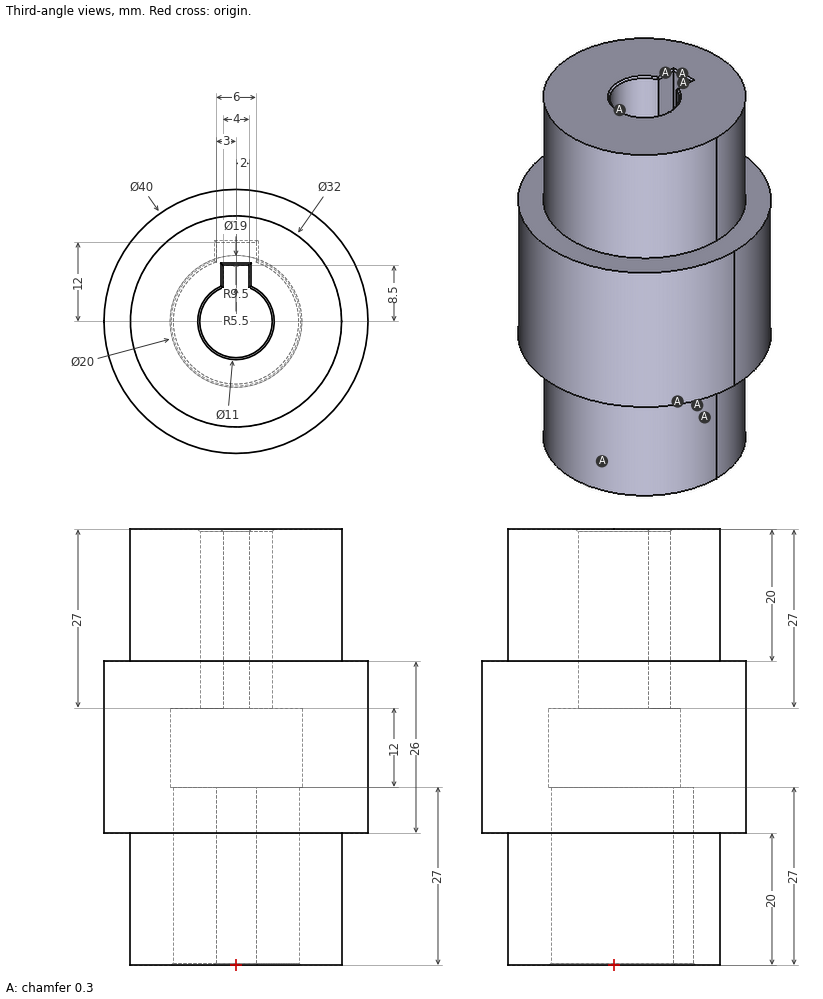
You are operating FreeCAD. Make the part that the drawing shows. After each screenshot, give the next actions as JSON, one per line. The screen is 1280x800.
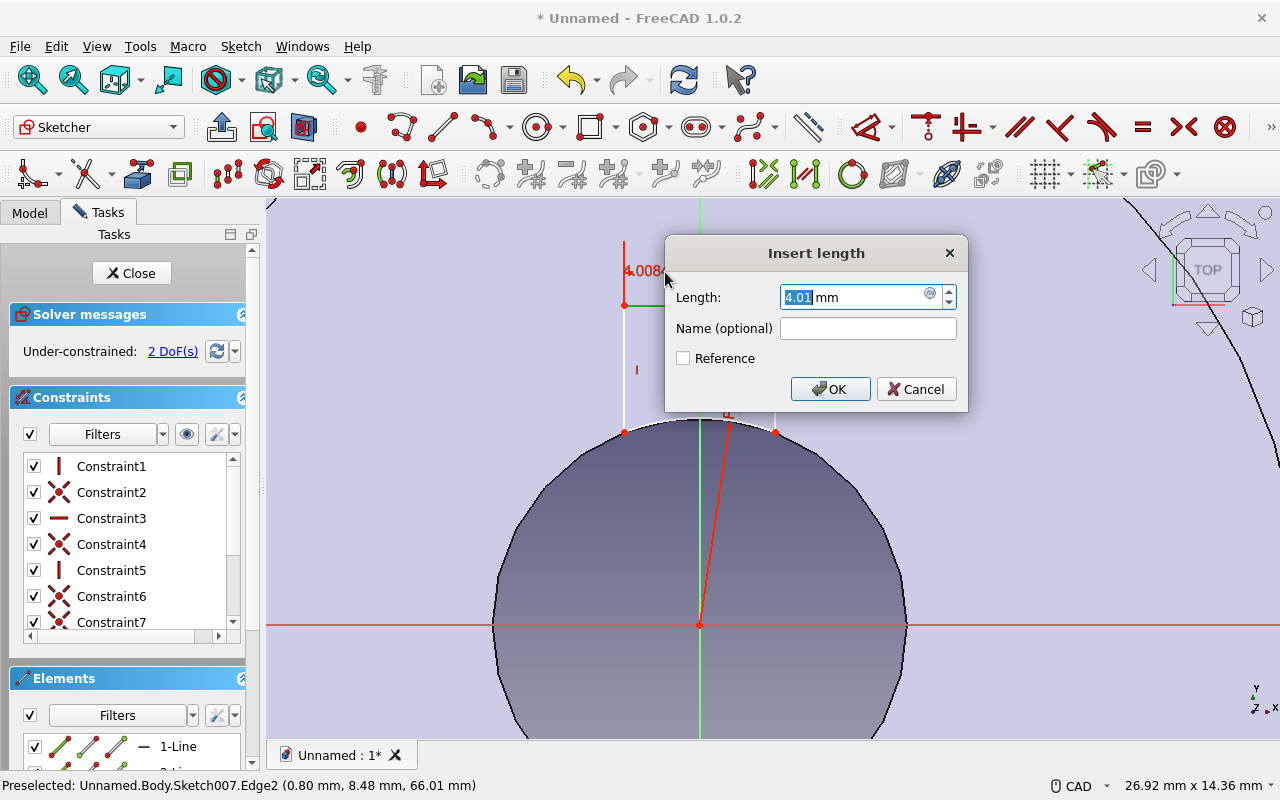
{"action": "type", "text": "4"}
{"action": "key", "text": "Return"}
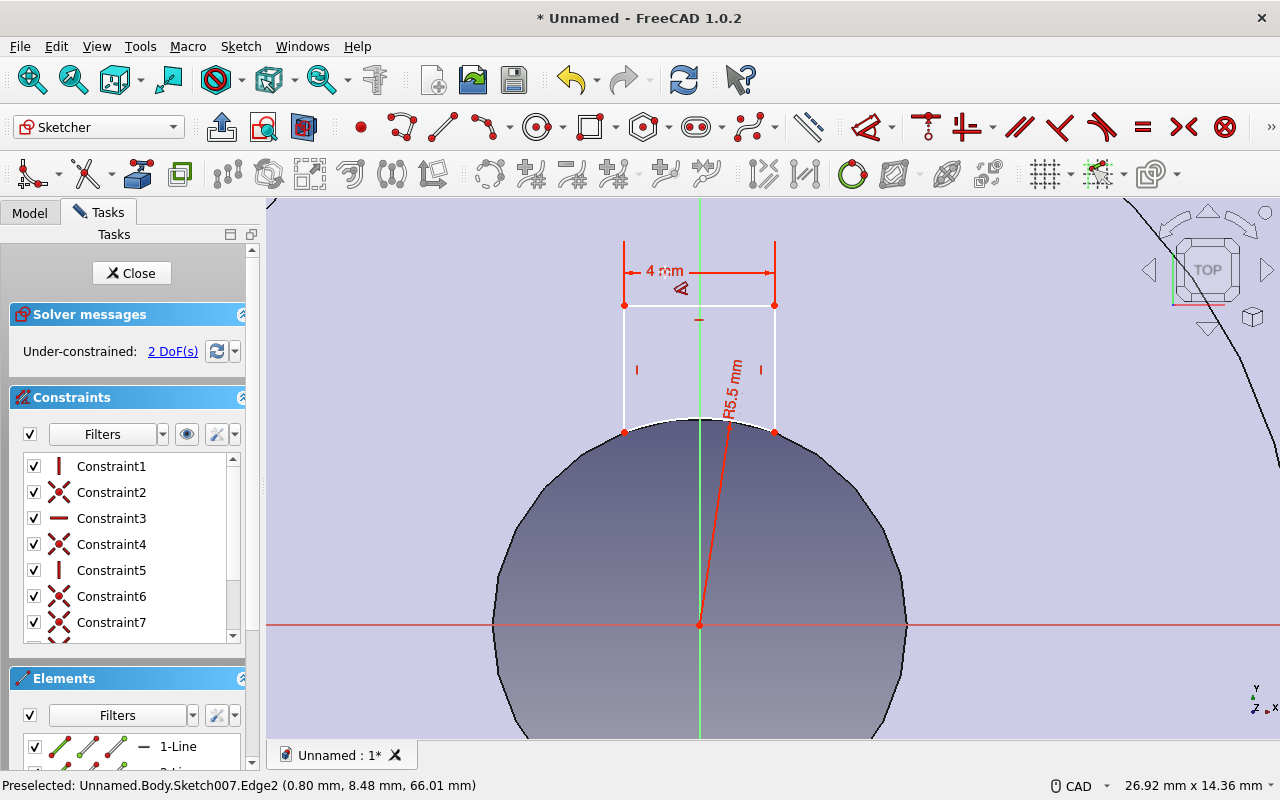
{"action": "left_click", "coordinate": [775, 432]}
{"action": "left_click", "coordinate": [737, 659]}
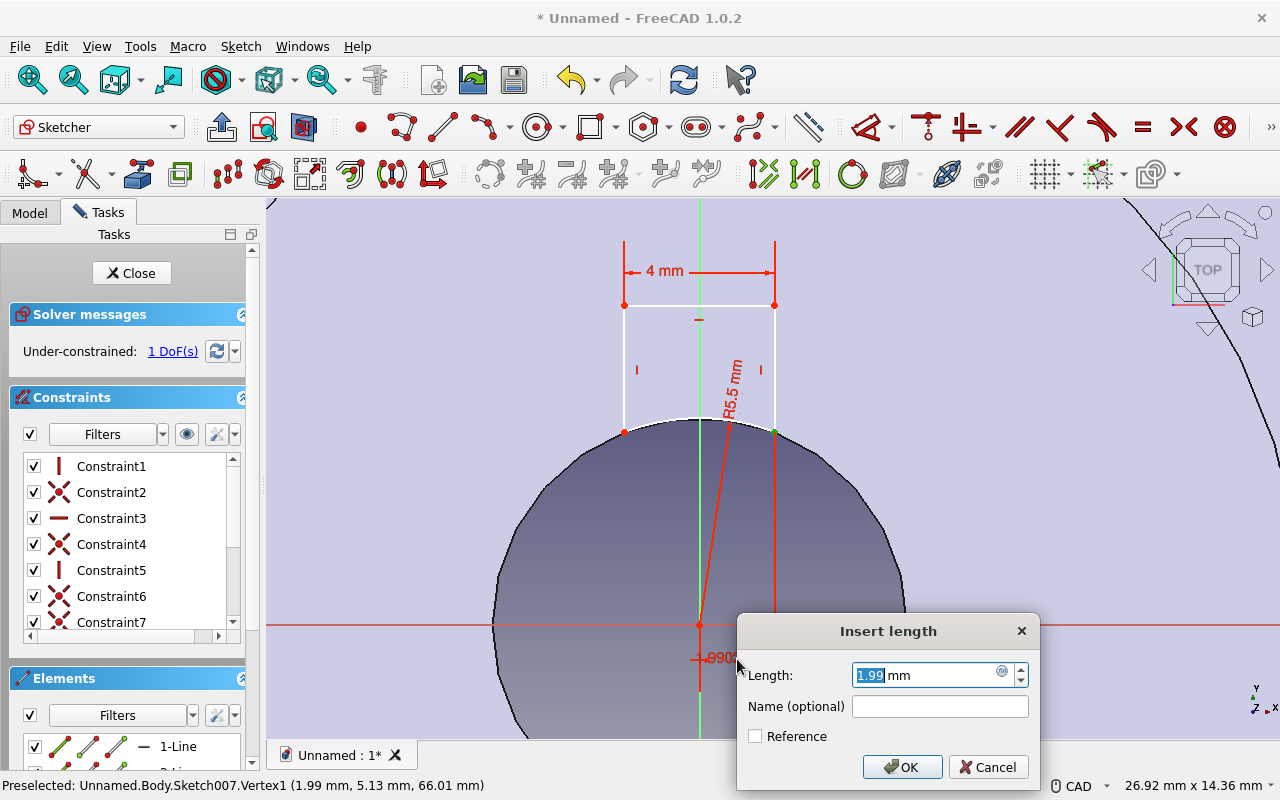
{"action": "type", "text": "2"}
{"action": "key", "text": "Return"}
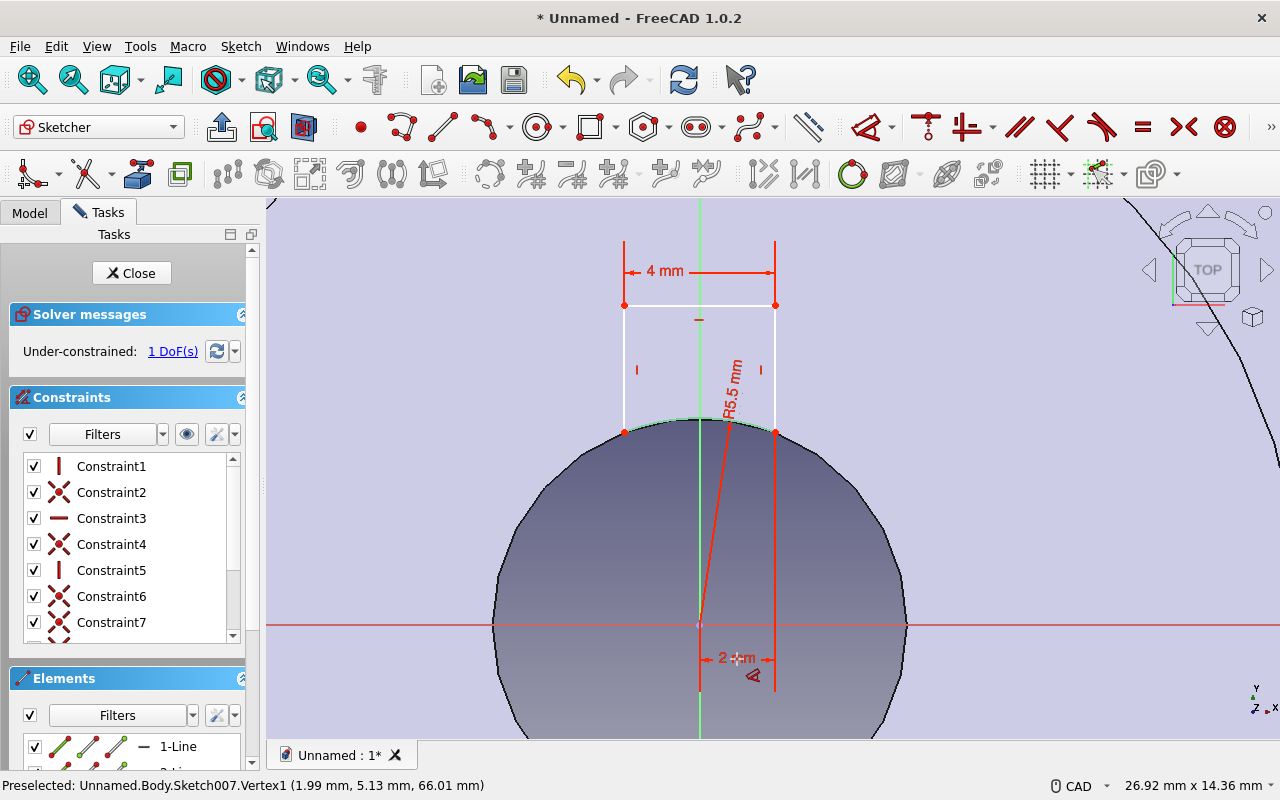
{"action": "left_click", "coordinate": [775, 306]}
{"action": "left_click", "coordinate": [809, 466]}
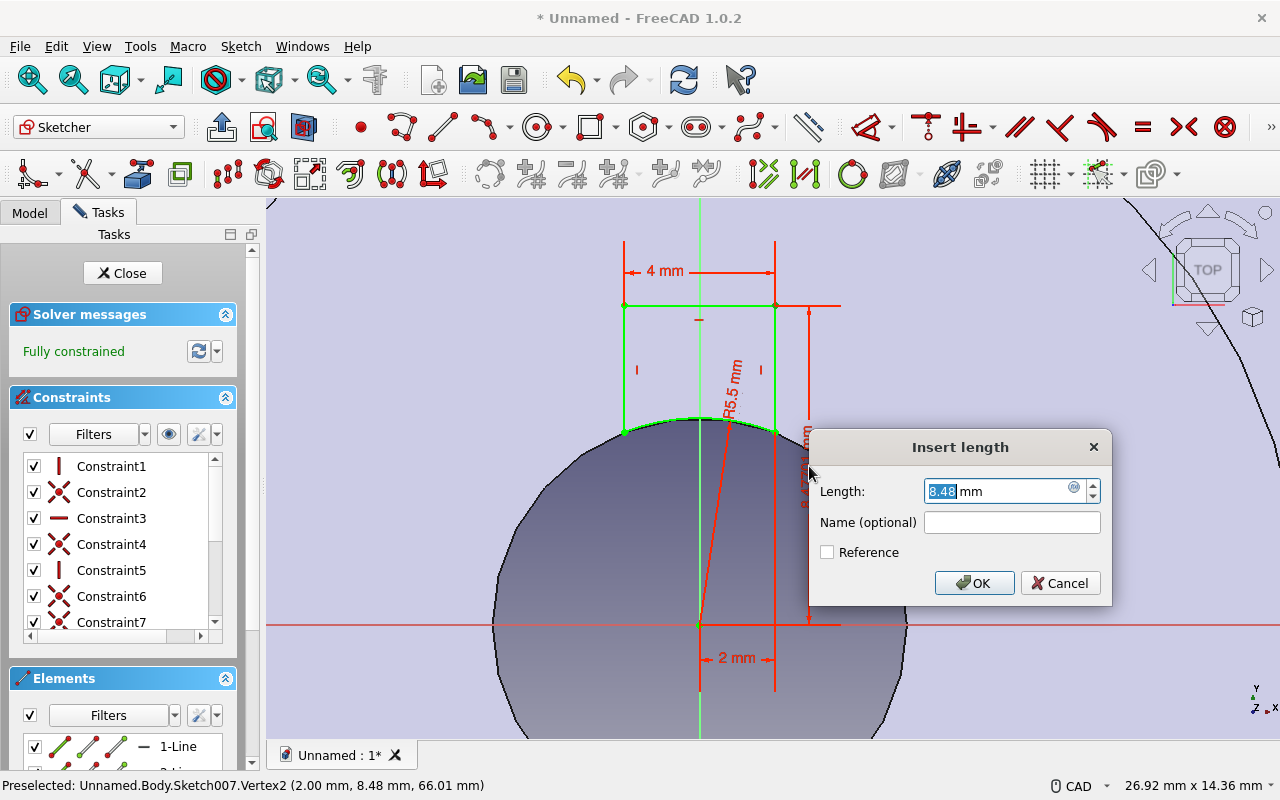
{"action": "type", "text": "8.5"}
{"action": "key", "text": "Return"}
{"action": "key", "text": "Escape"}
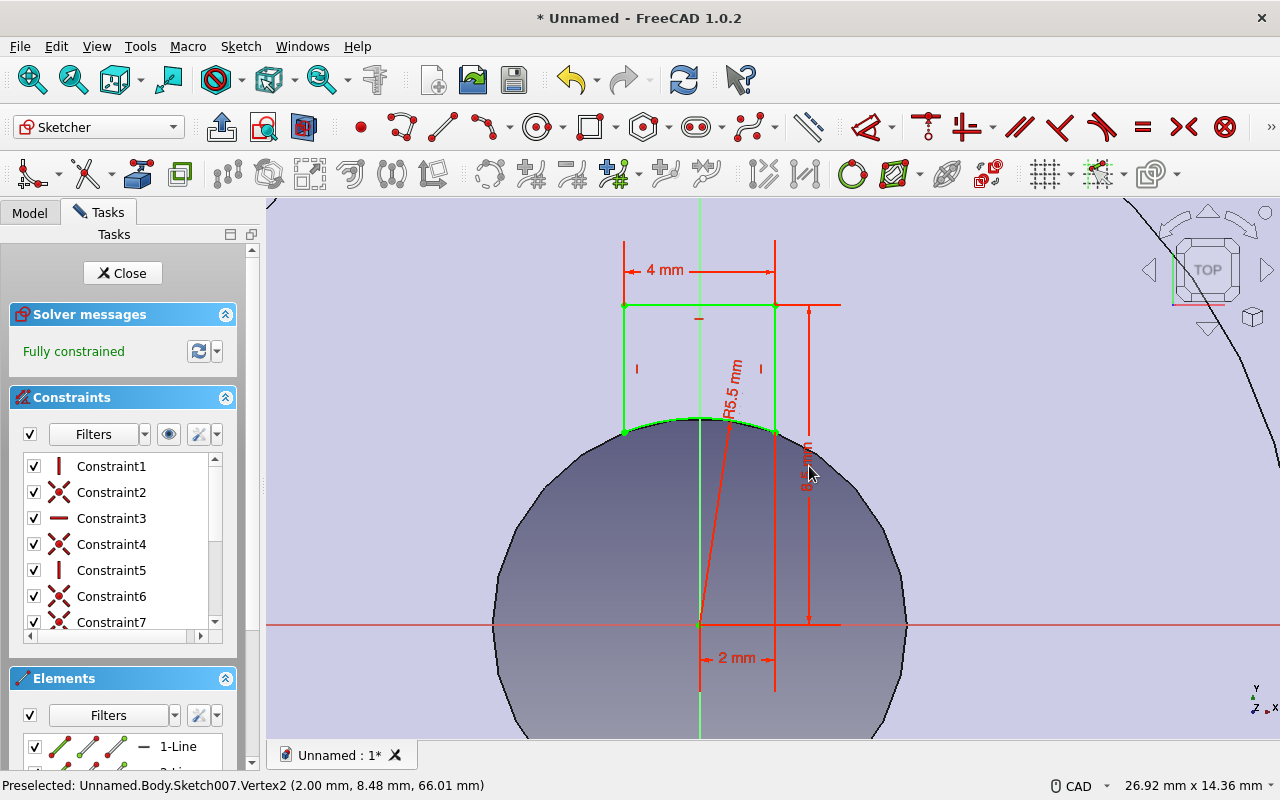
{"action": "left_click", "coordinate": [123, 273]}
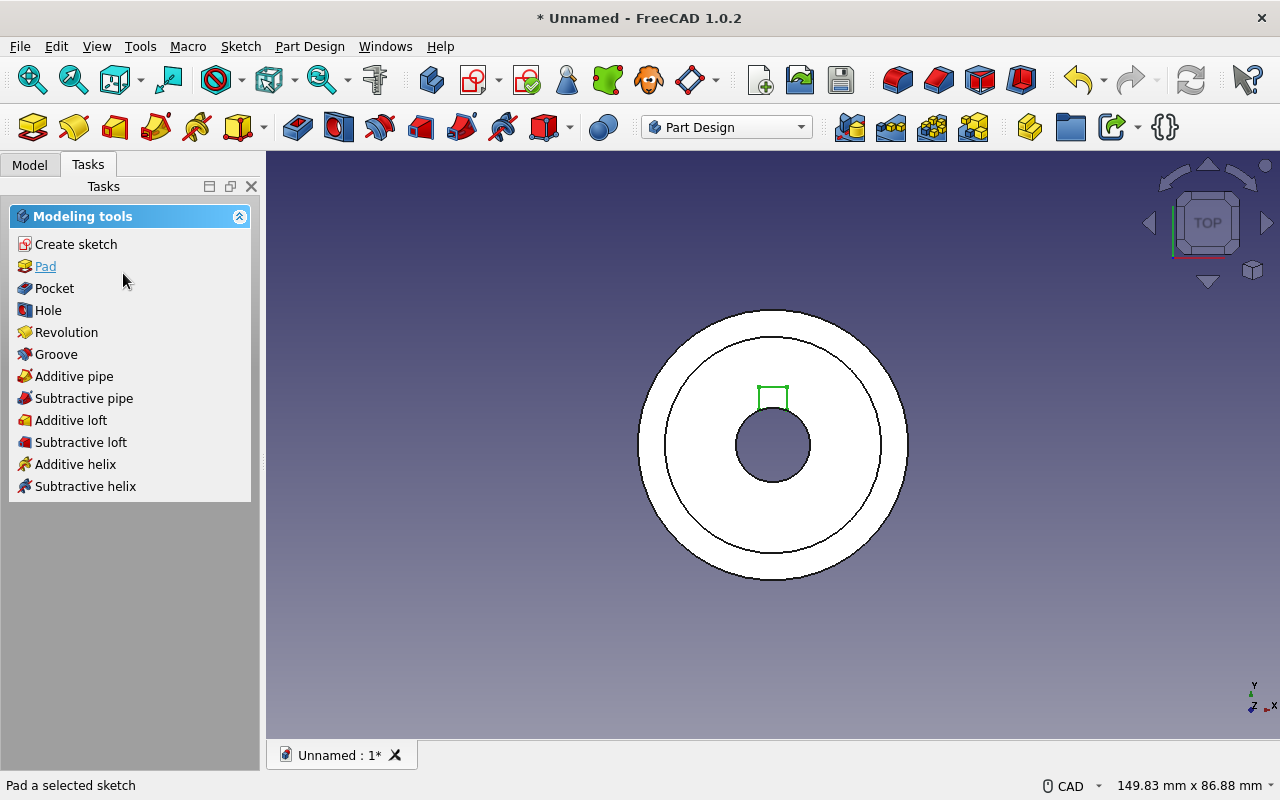
{"action": "left_click", "coordinate": [298, 128]}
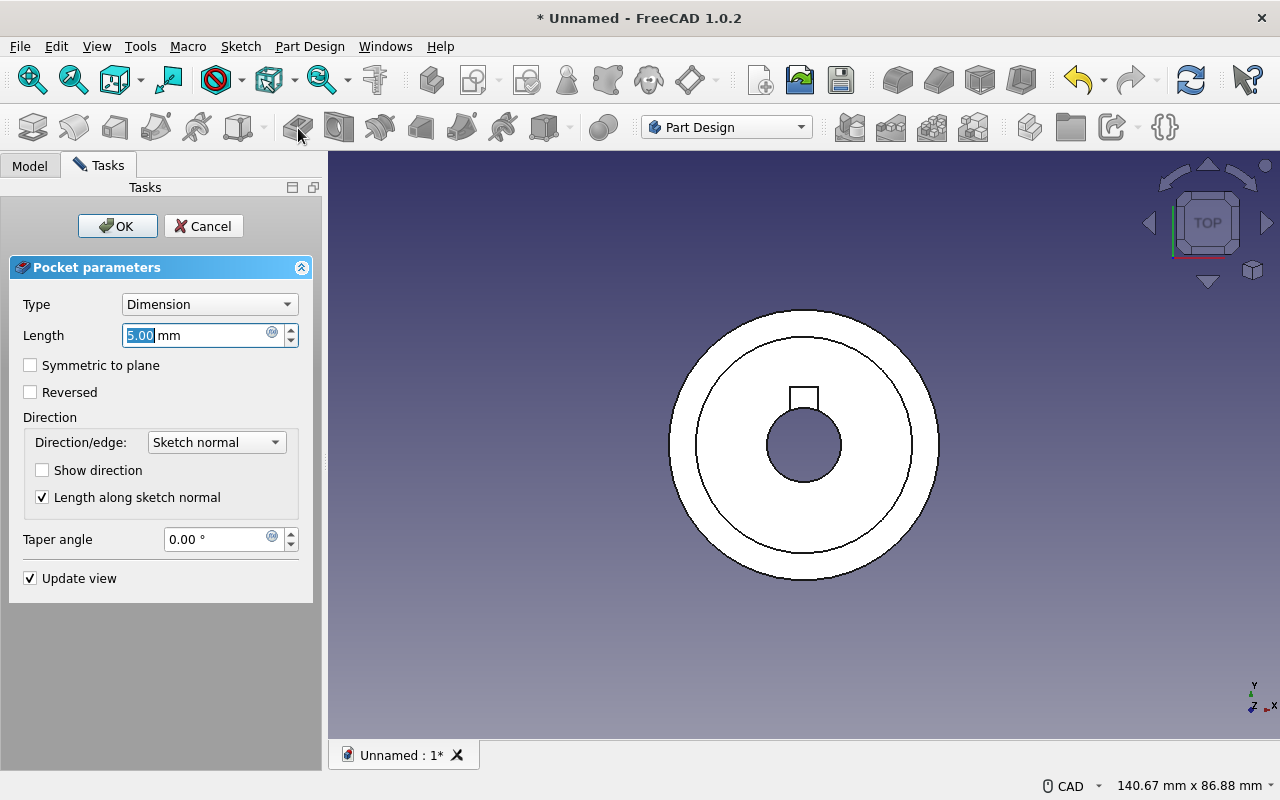
{"action": "type", "text": "27"}
{"action": "key", "text": "Tab"}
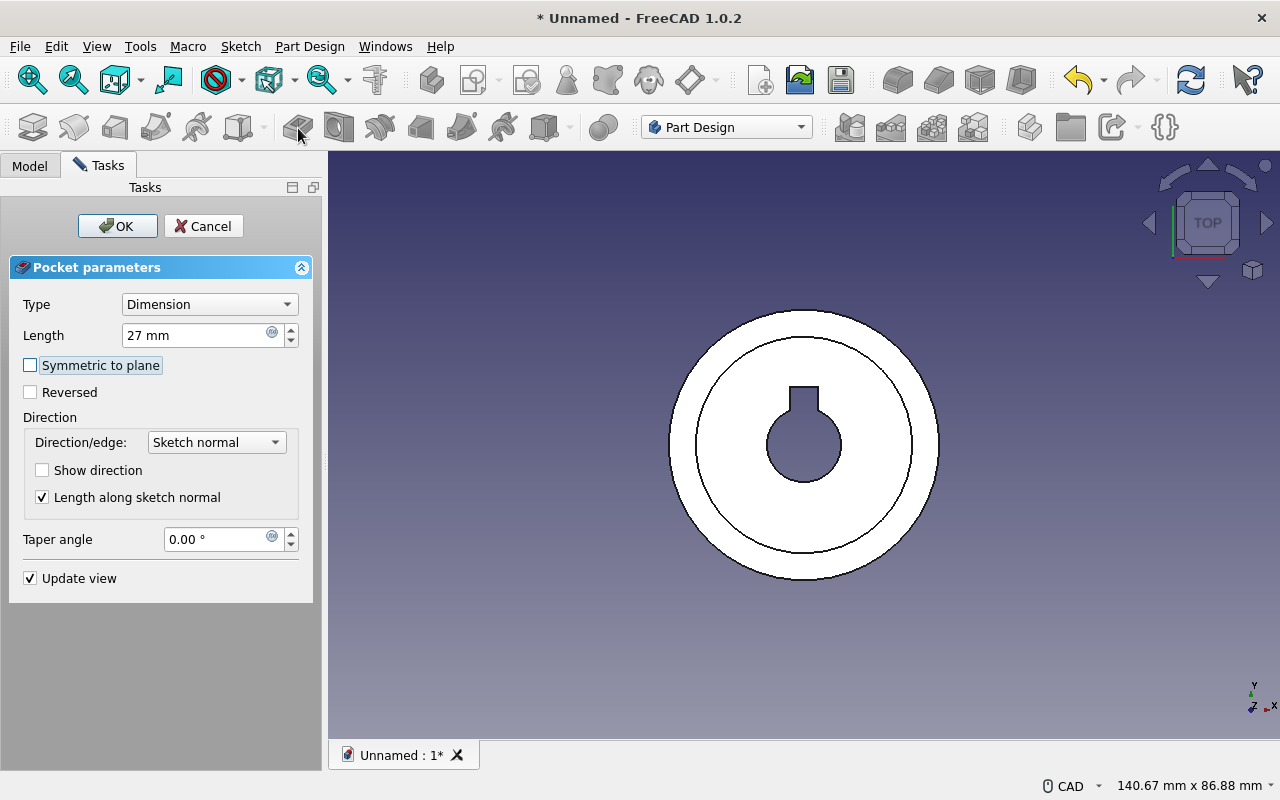
{"action": "left_click", "coordinate": [118, 226]}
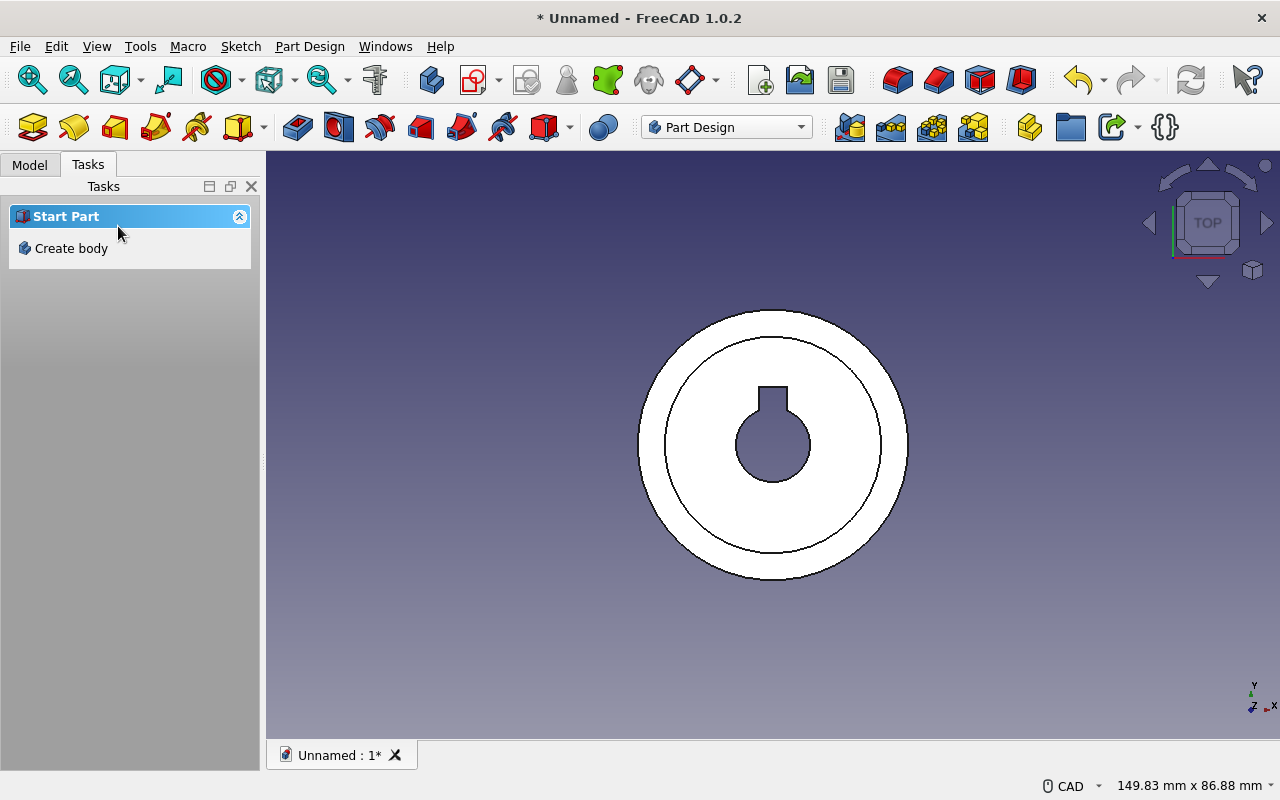
{"action": "left_click", "coordinate": [752, 475]}